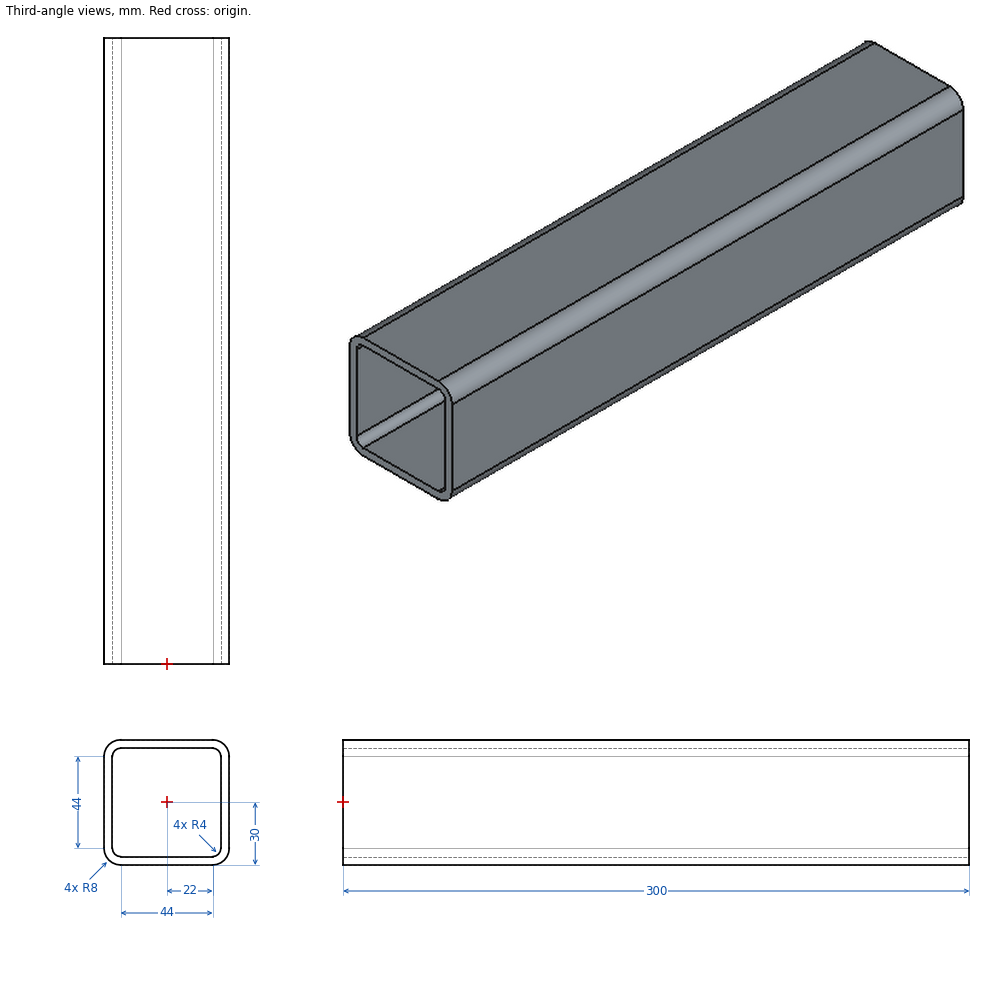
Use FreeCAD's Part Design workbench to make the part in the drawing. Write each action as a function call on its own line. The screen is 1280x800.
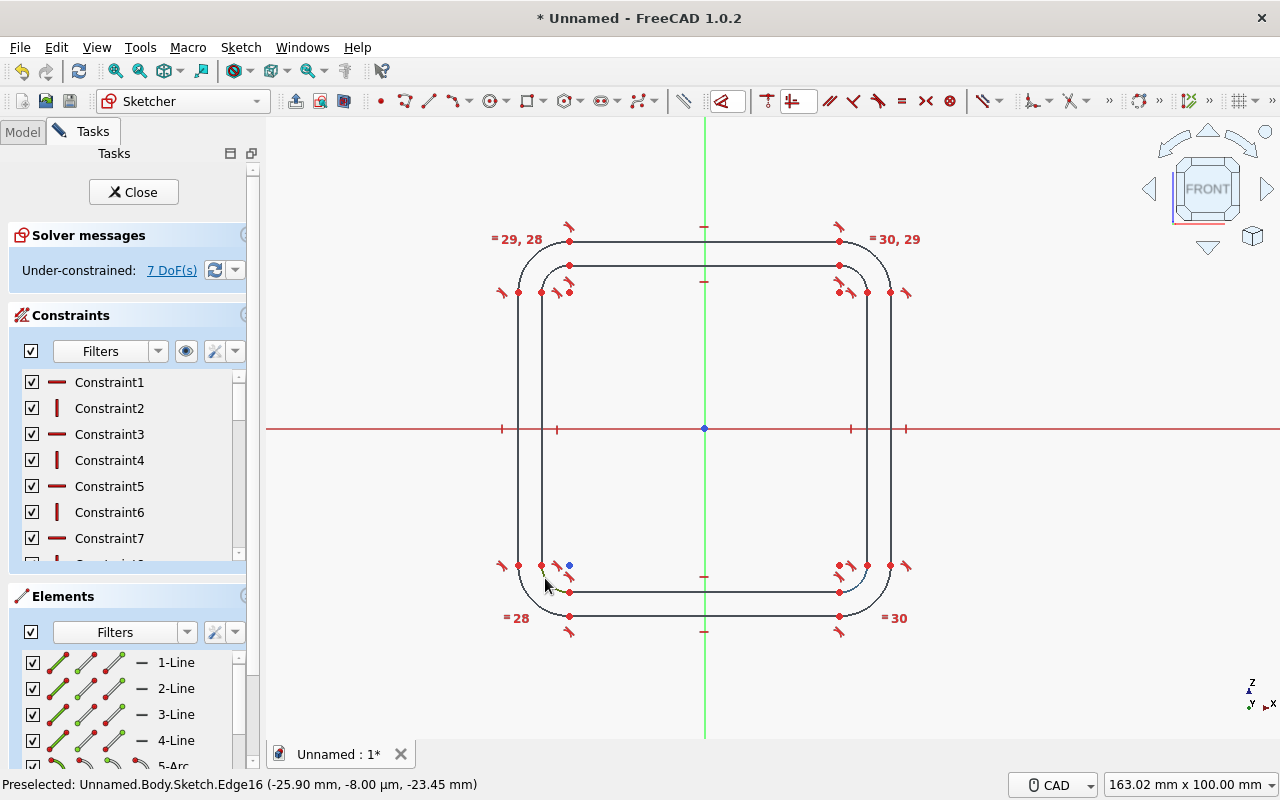
key(e)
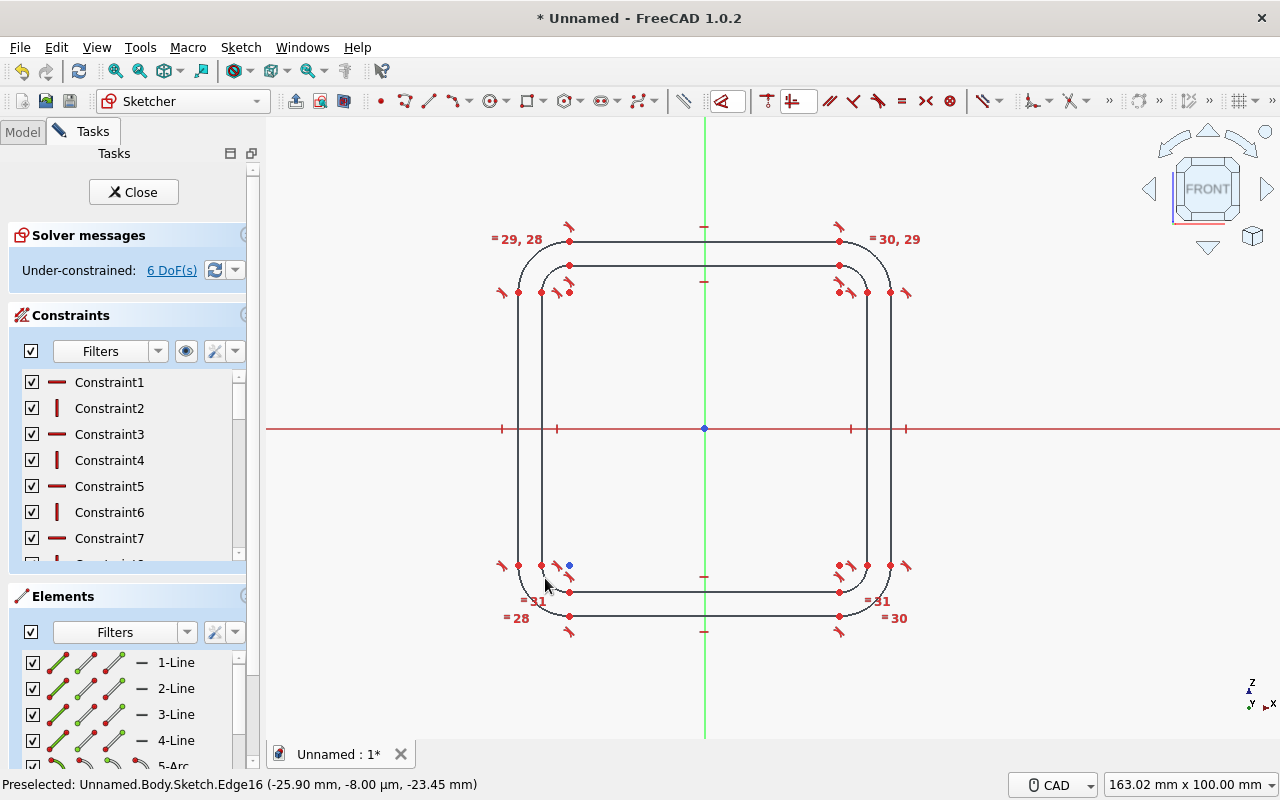
key(d)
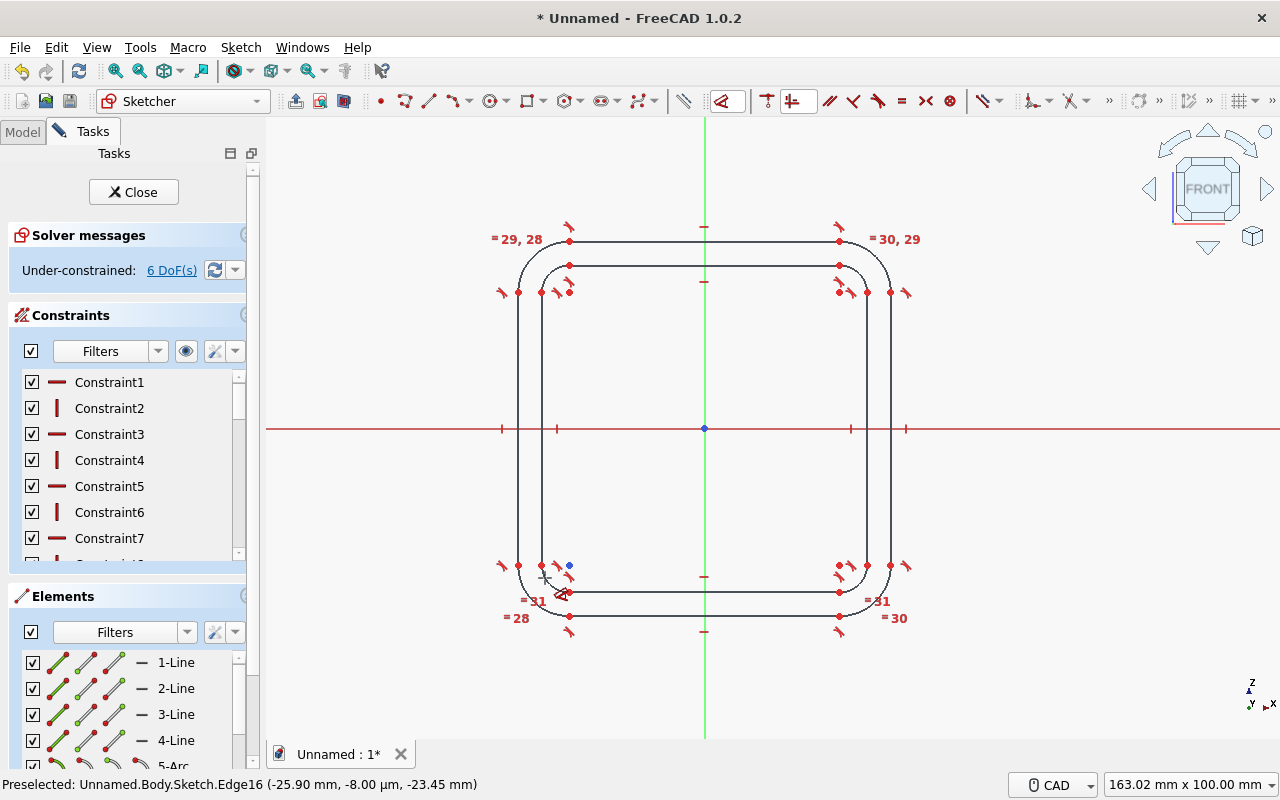
click(524, 588)
click(495, 602)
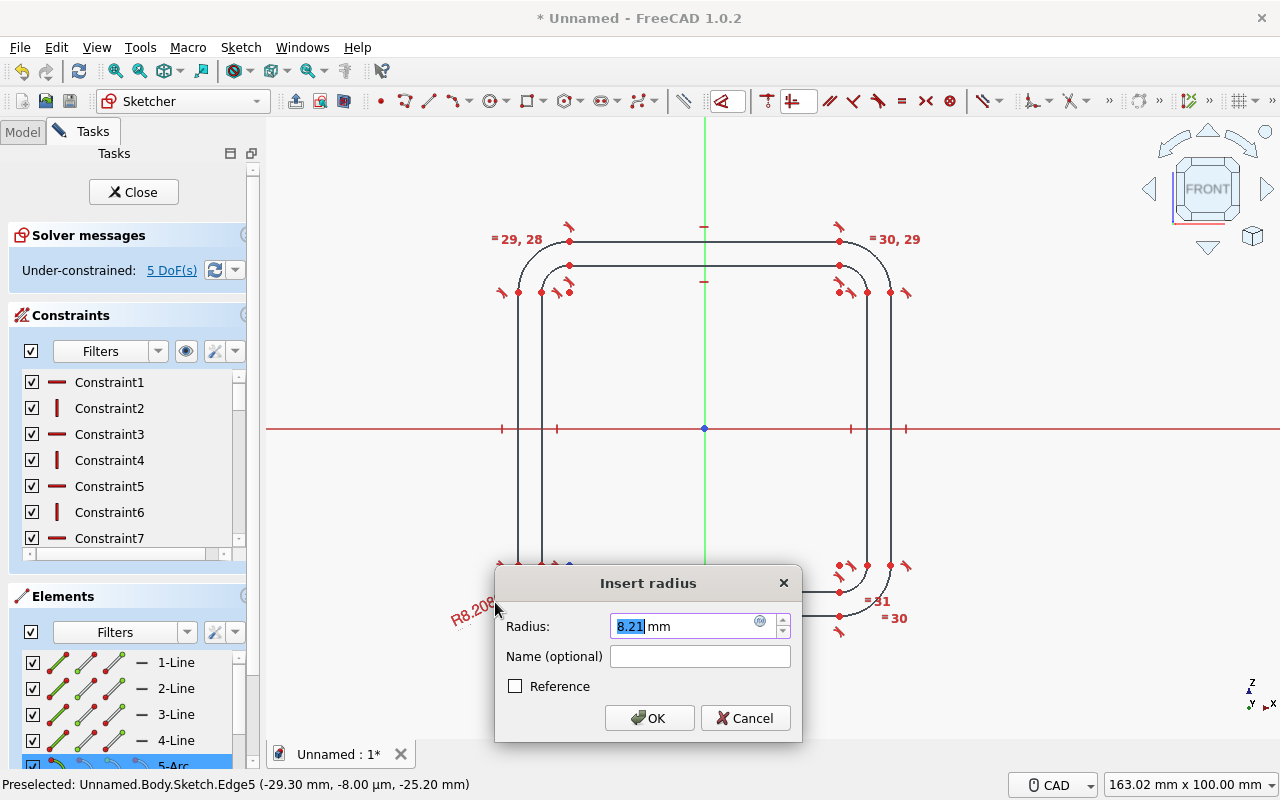
text(8)
key(Return)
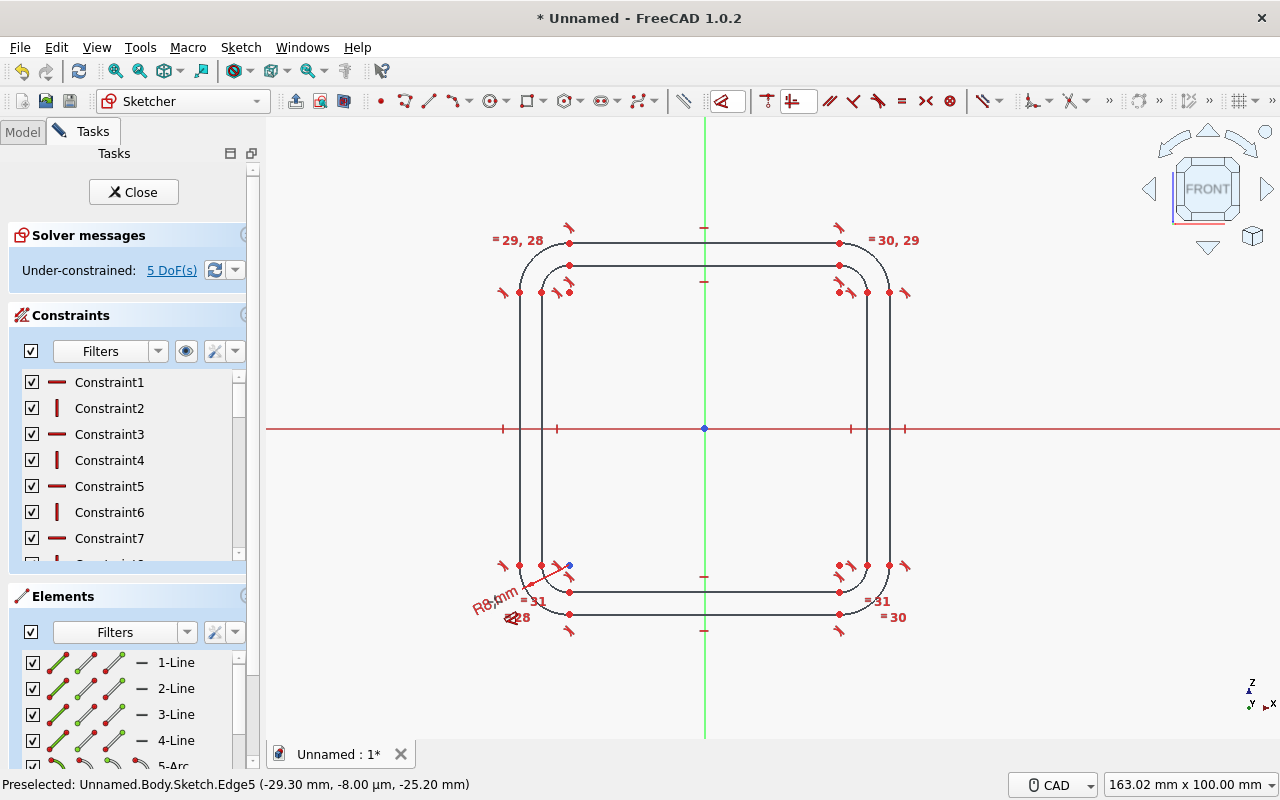
scroll(852, 589, up, 3)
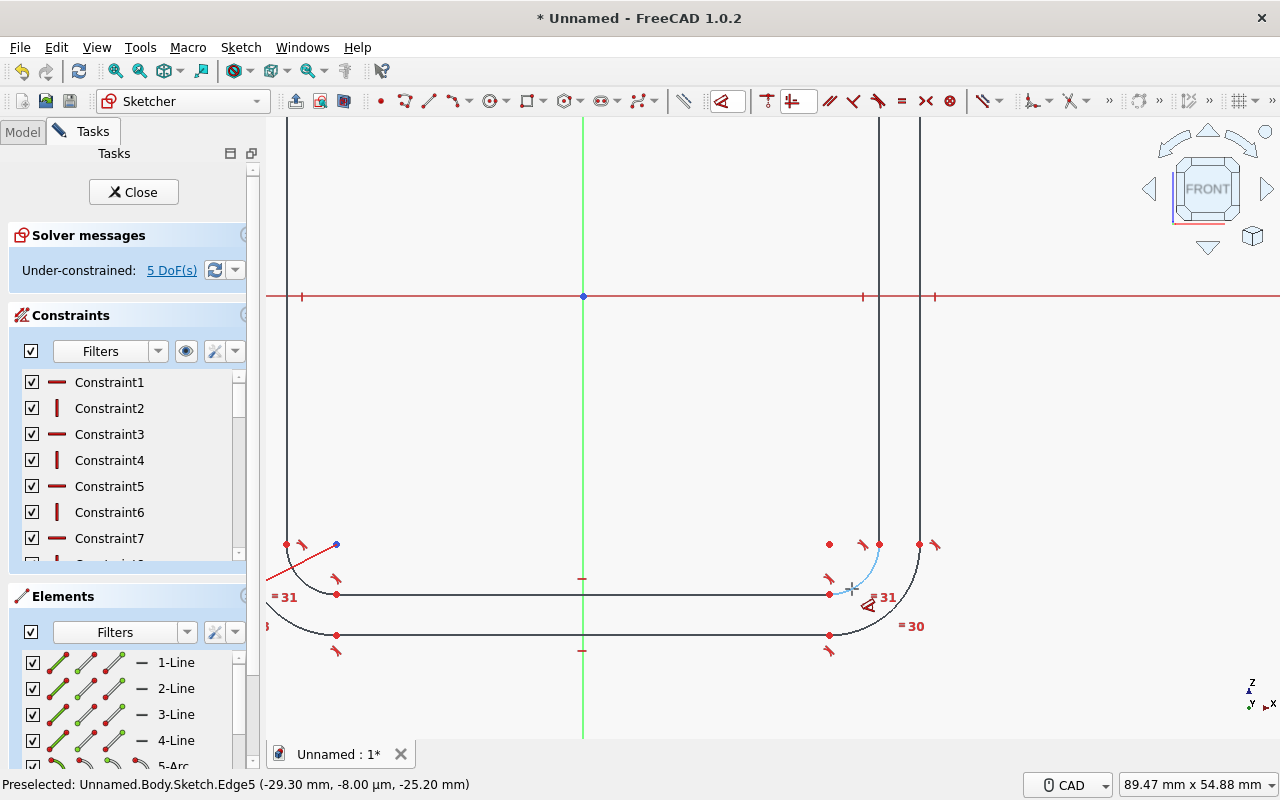
click(852, 589)
click(788, 616)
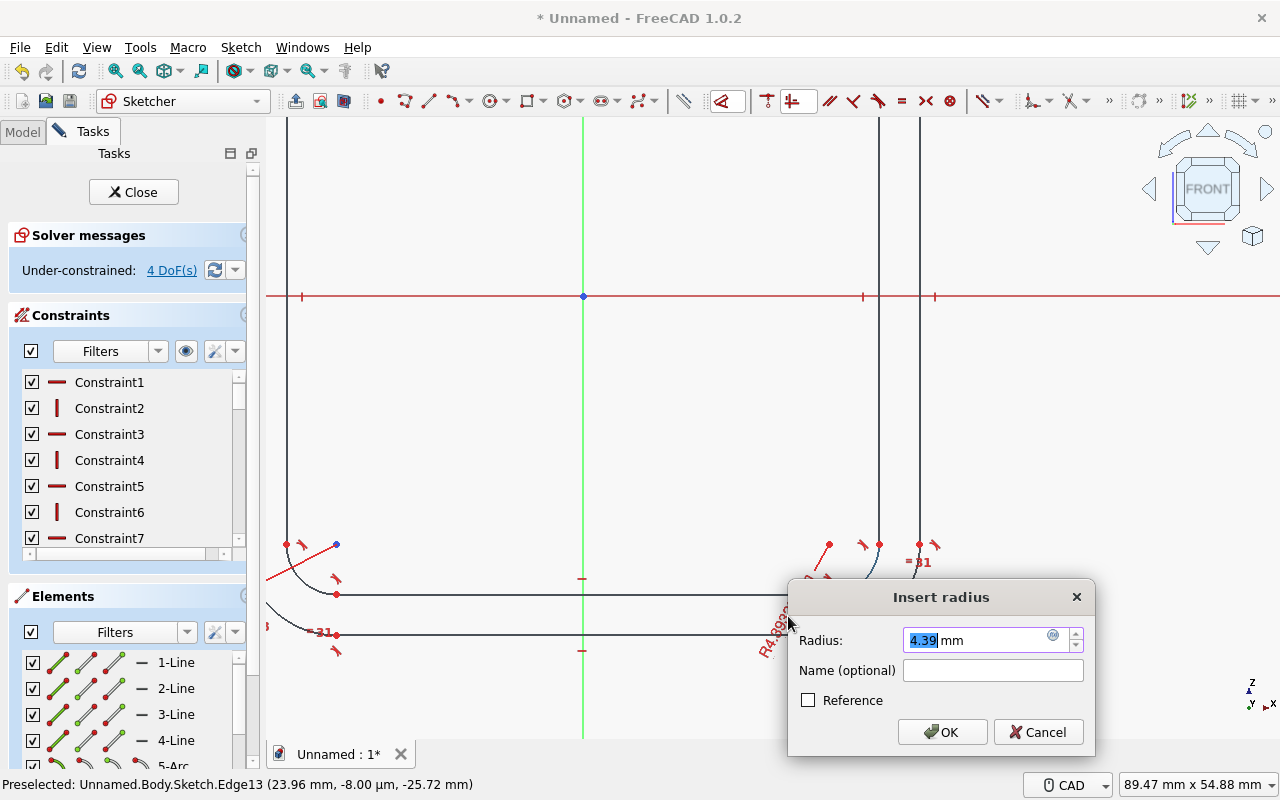
text(4)
key(Return)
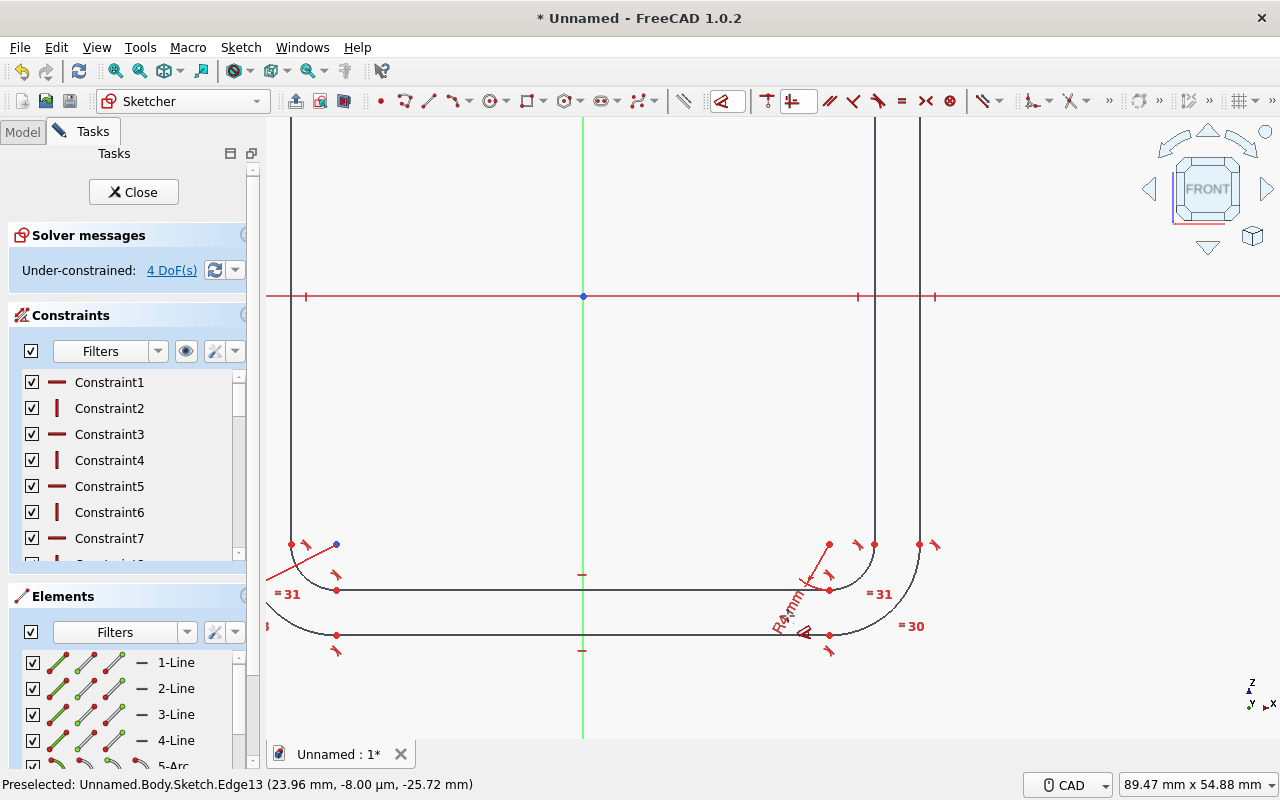
click(681, 635)
click(469, 669)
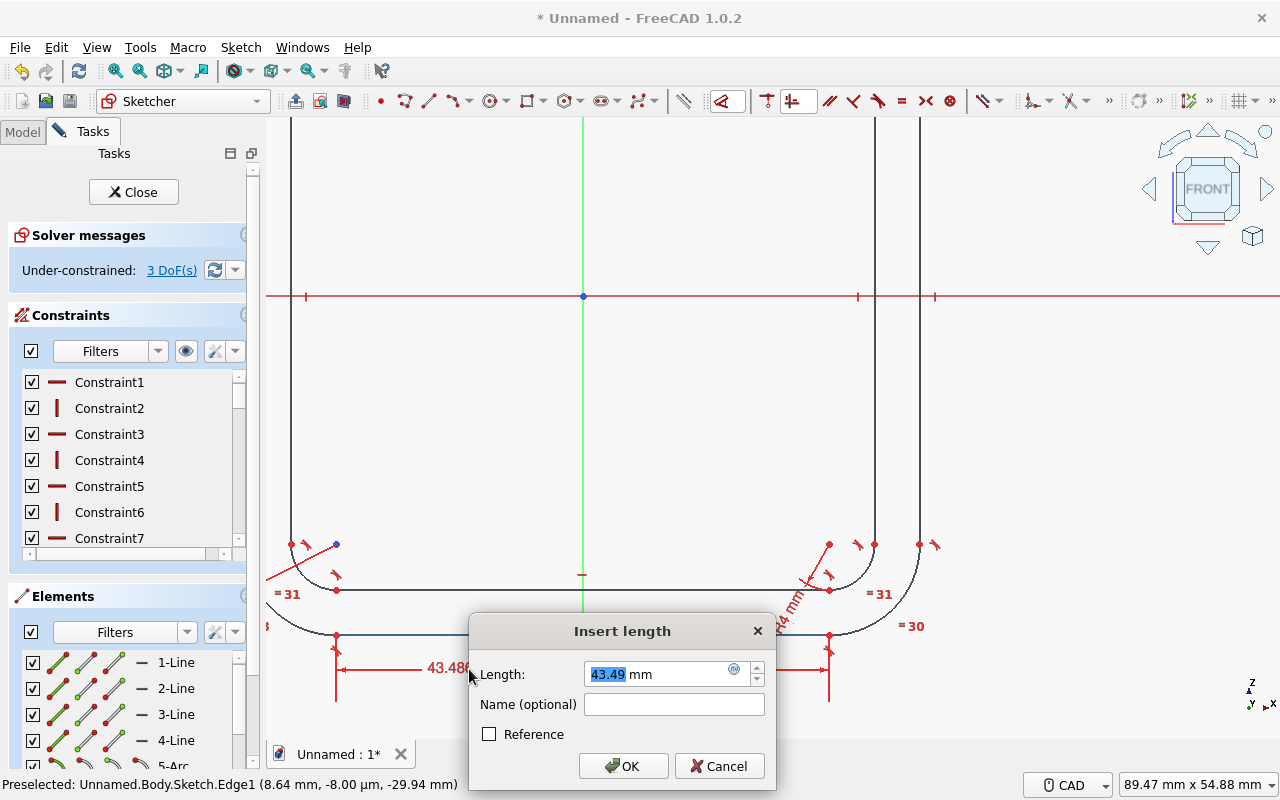
text(44)
key(Return)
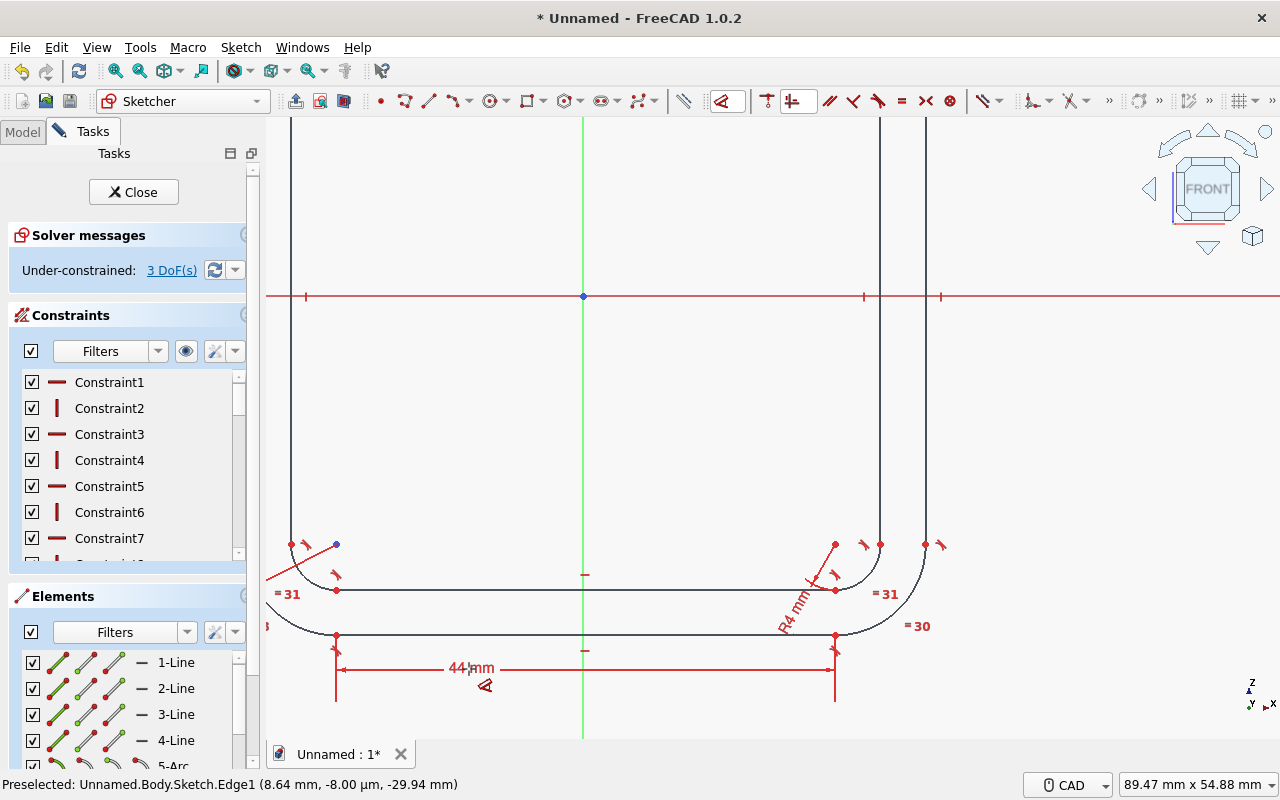
scroll(852, 589, down, 3)